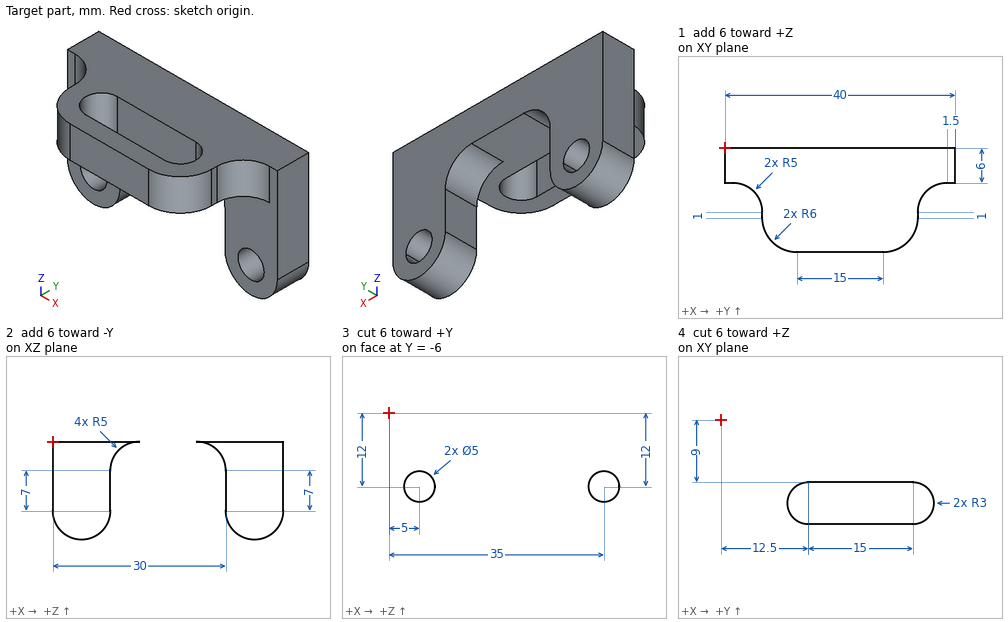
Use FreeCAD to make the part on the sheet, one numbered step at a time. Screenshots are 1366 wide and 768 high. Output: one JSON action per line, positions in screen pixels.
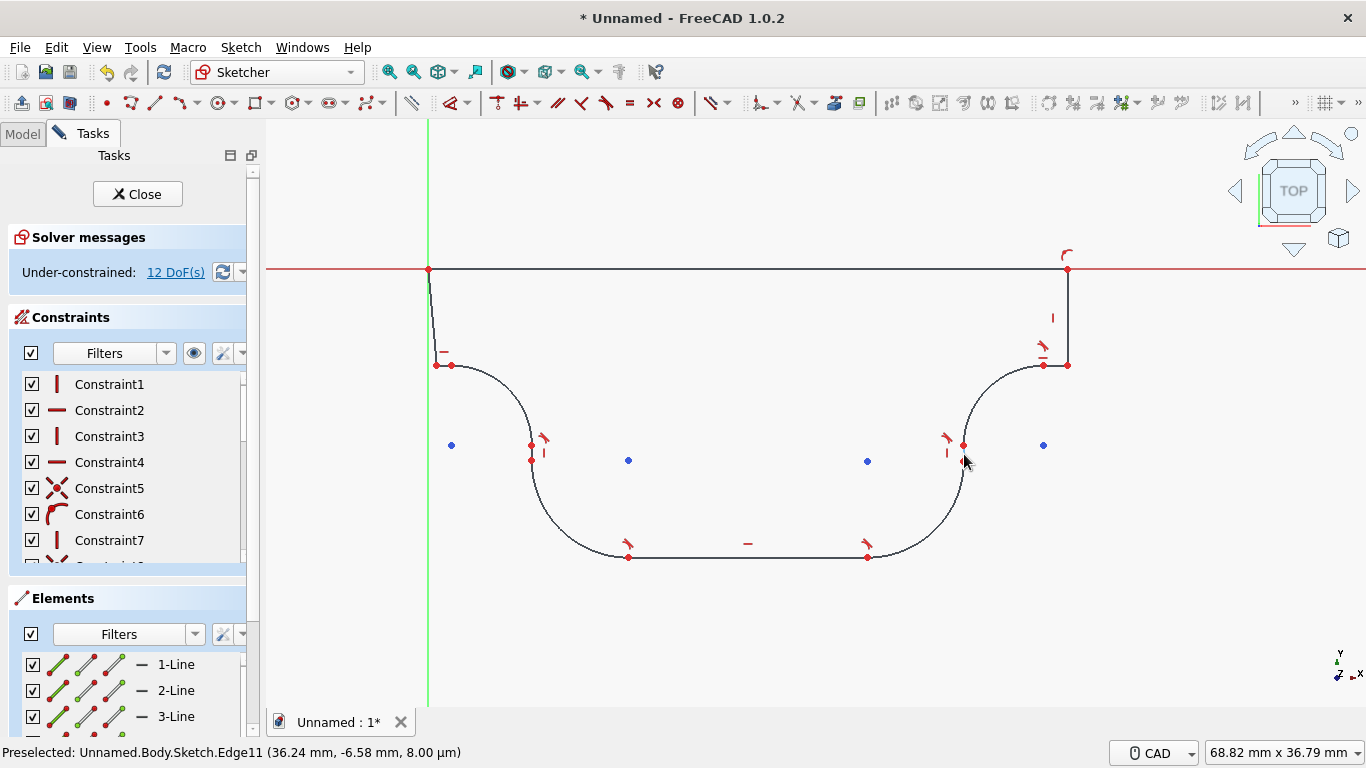
{"action": "scroll", "coordinate": [441, 366], "scroll_direction": "up", "scroll_amount": 6}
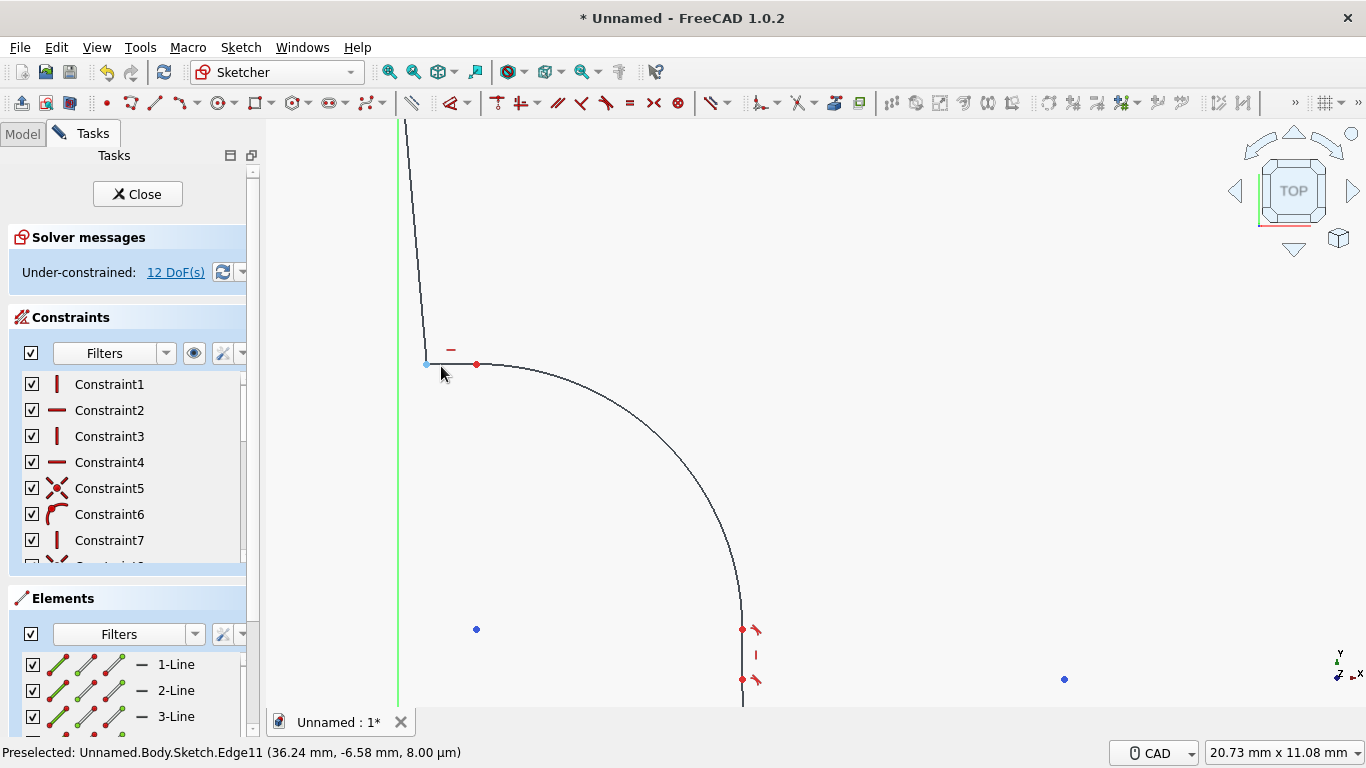
{"action": "left_click", "coordinate": [442, 364]}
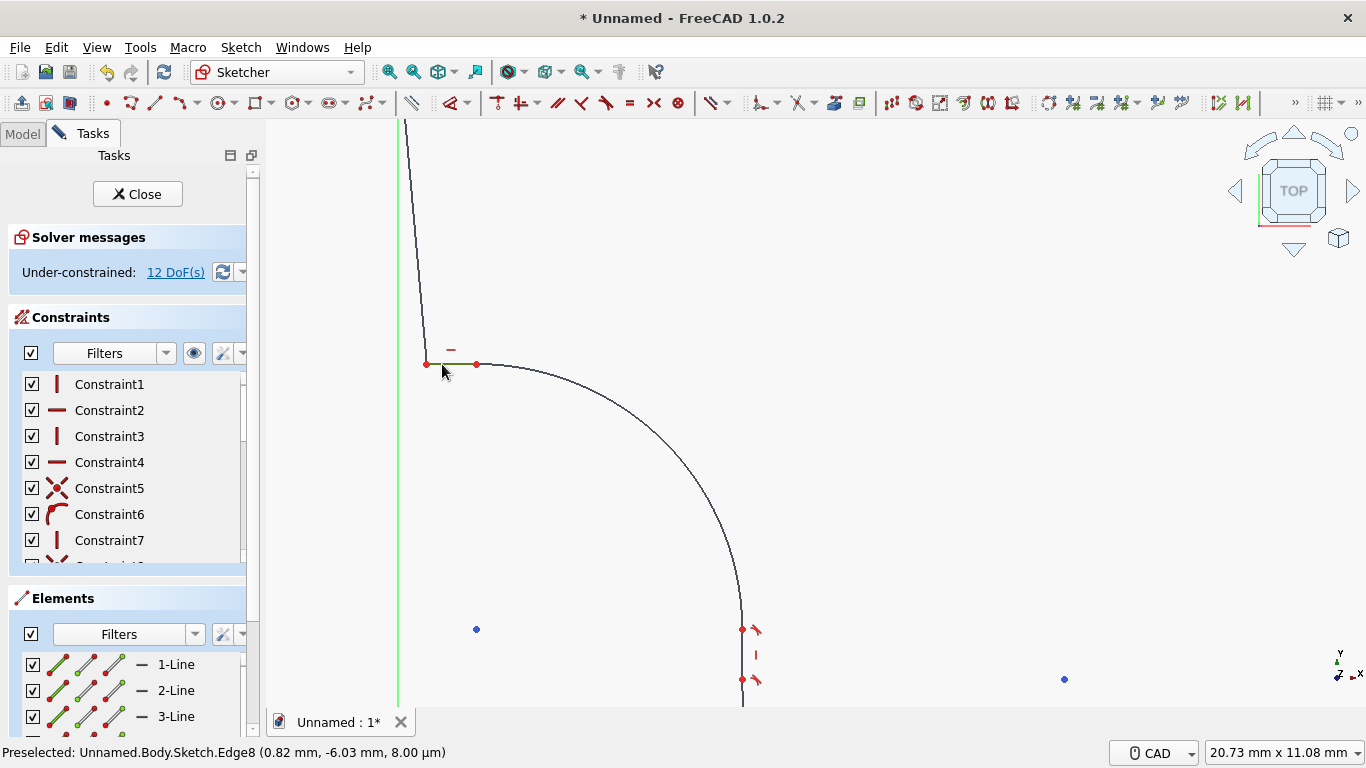
{"action": "left_click", "coordinate": [713, 509]}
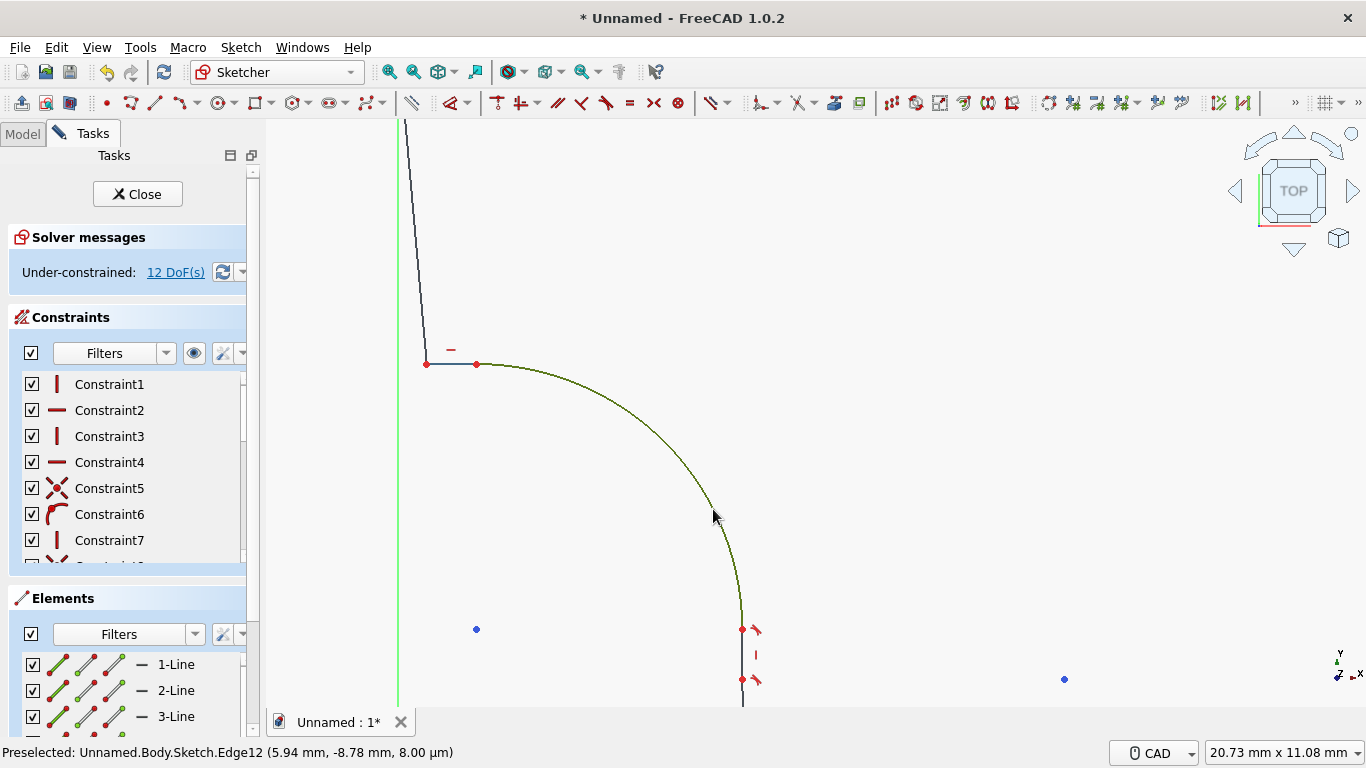
{"action": "left_click", "coordinate": [606, 104]}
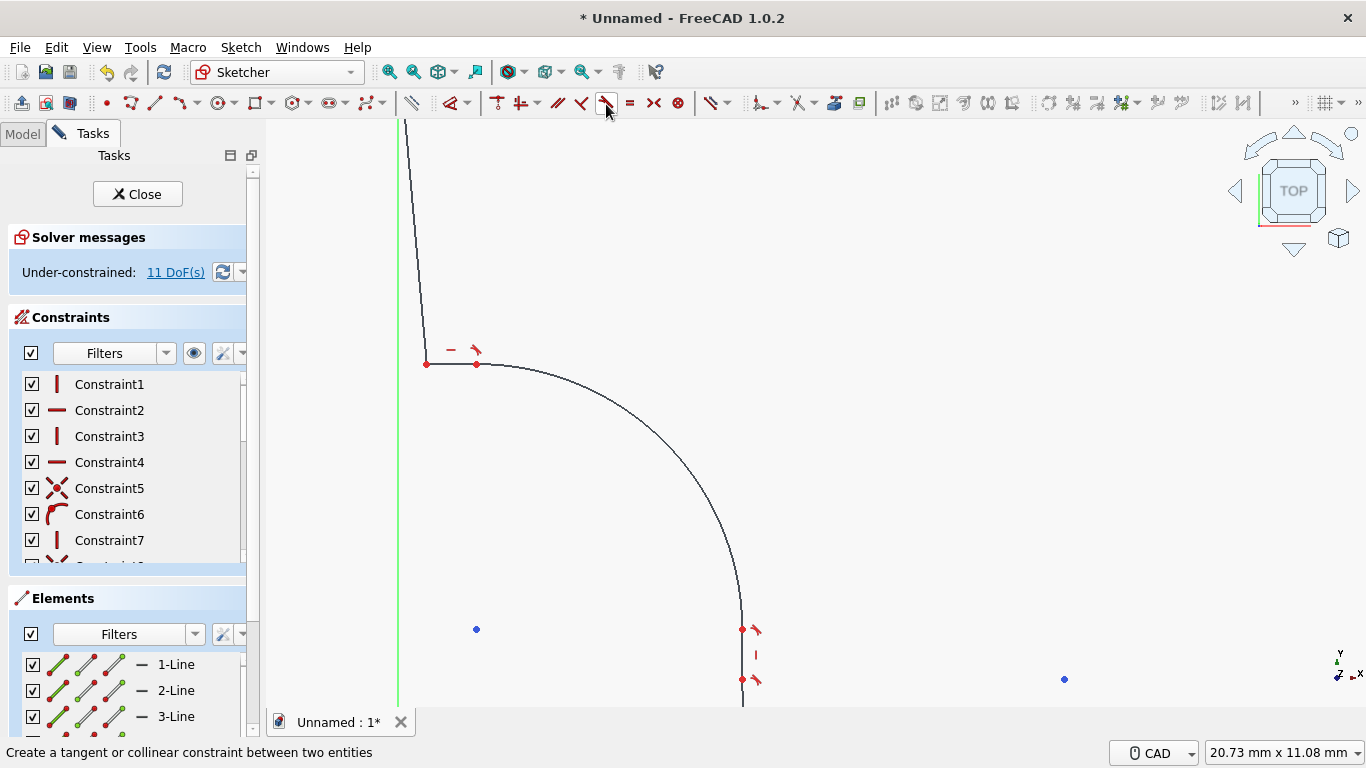
{"action": "left_click", "coordinate": [418, 268]}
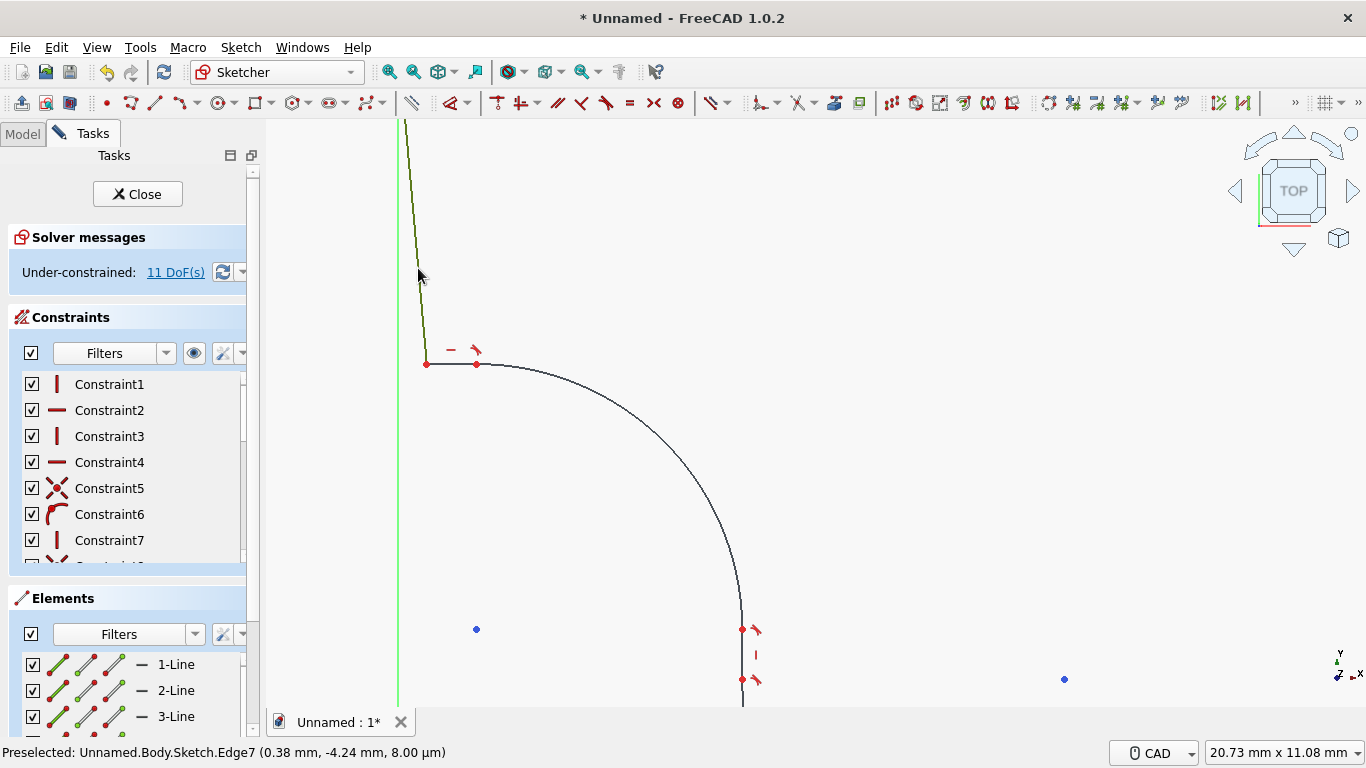
{"action": "key", "text": "v"}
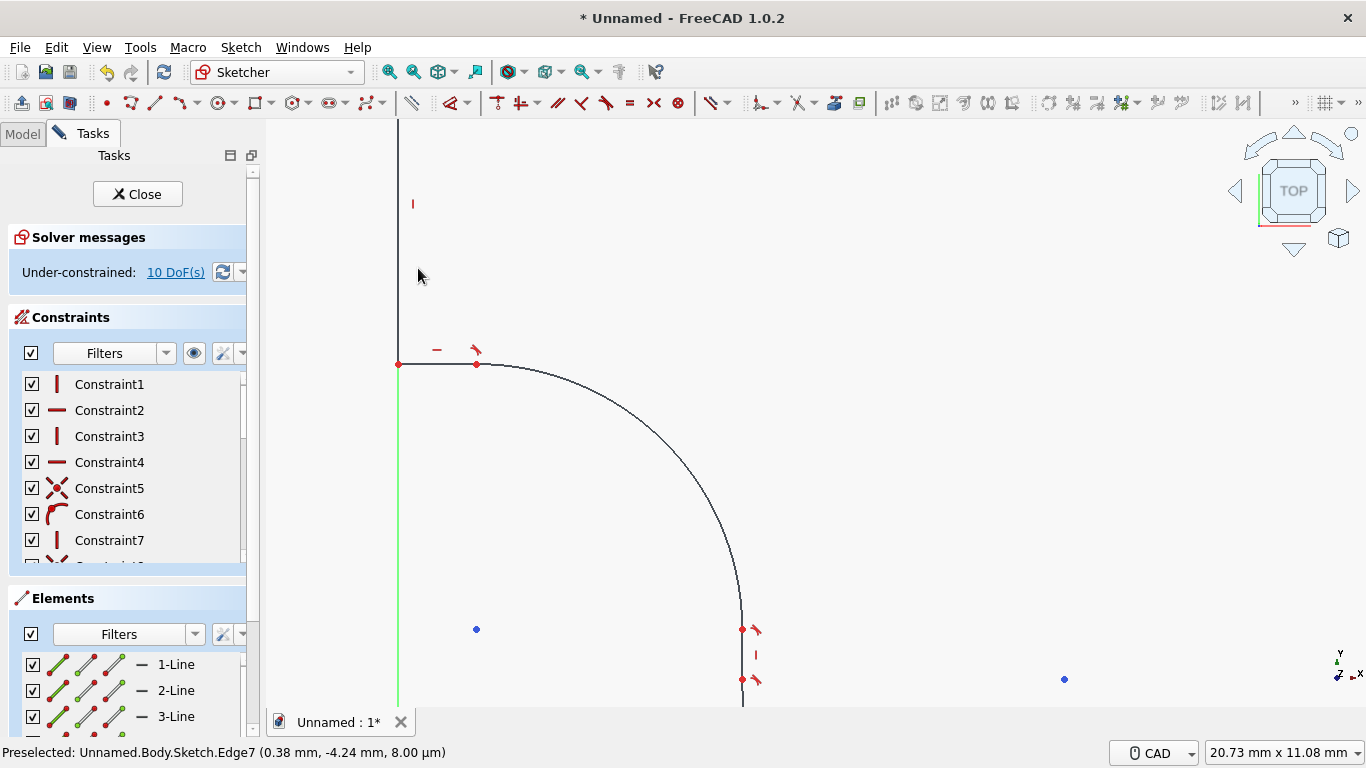
{"action": "scroll", "coordinate": [441, 366], "scroll_direction": "down", "scroll_amount": 6}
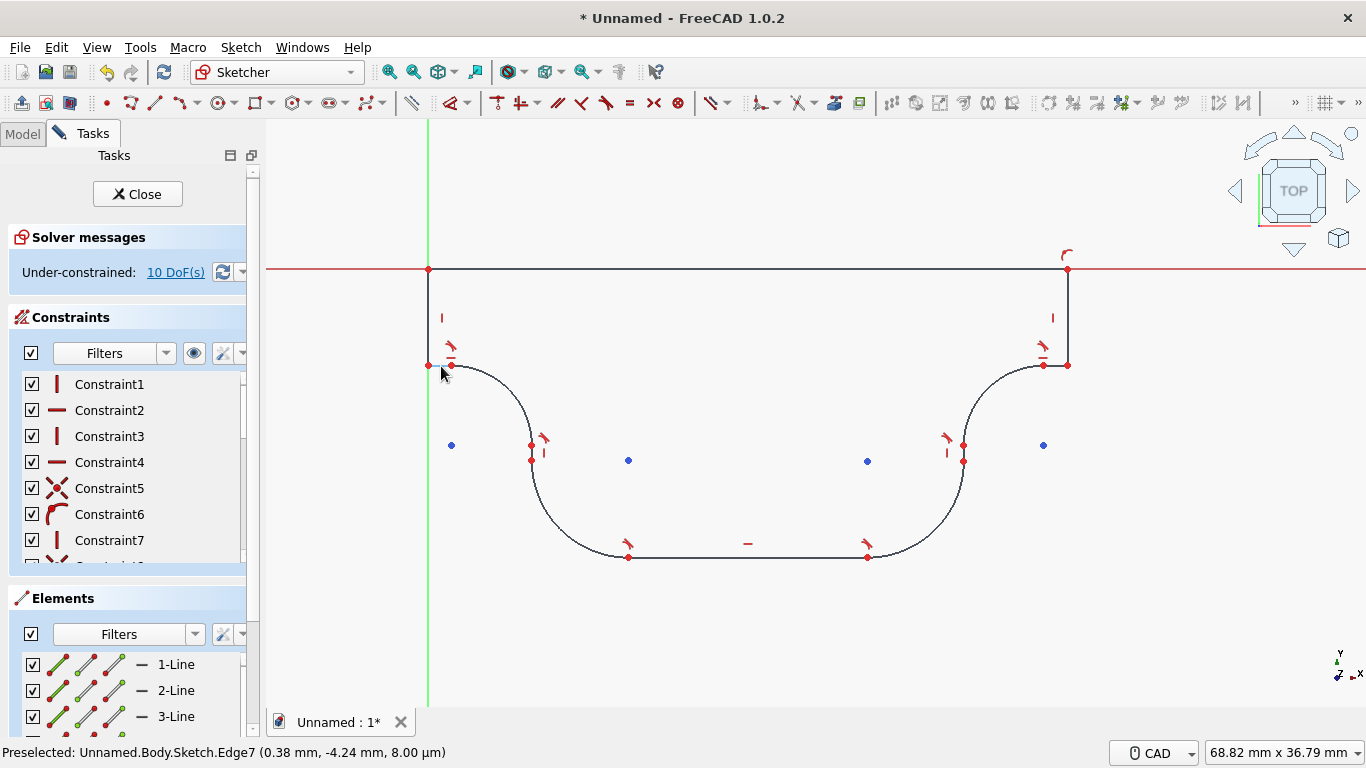
{"action": "left_click", "coordinate": [542, 505]}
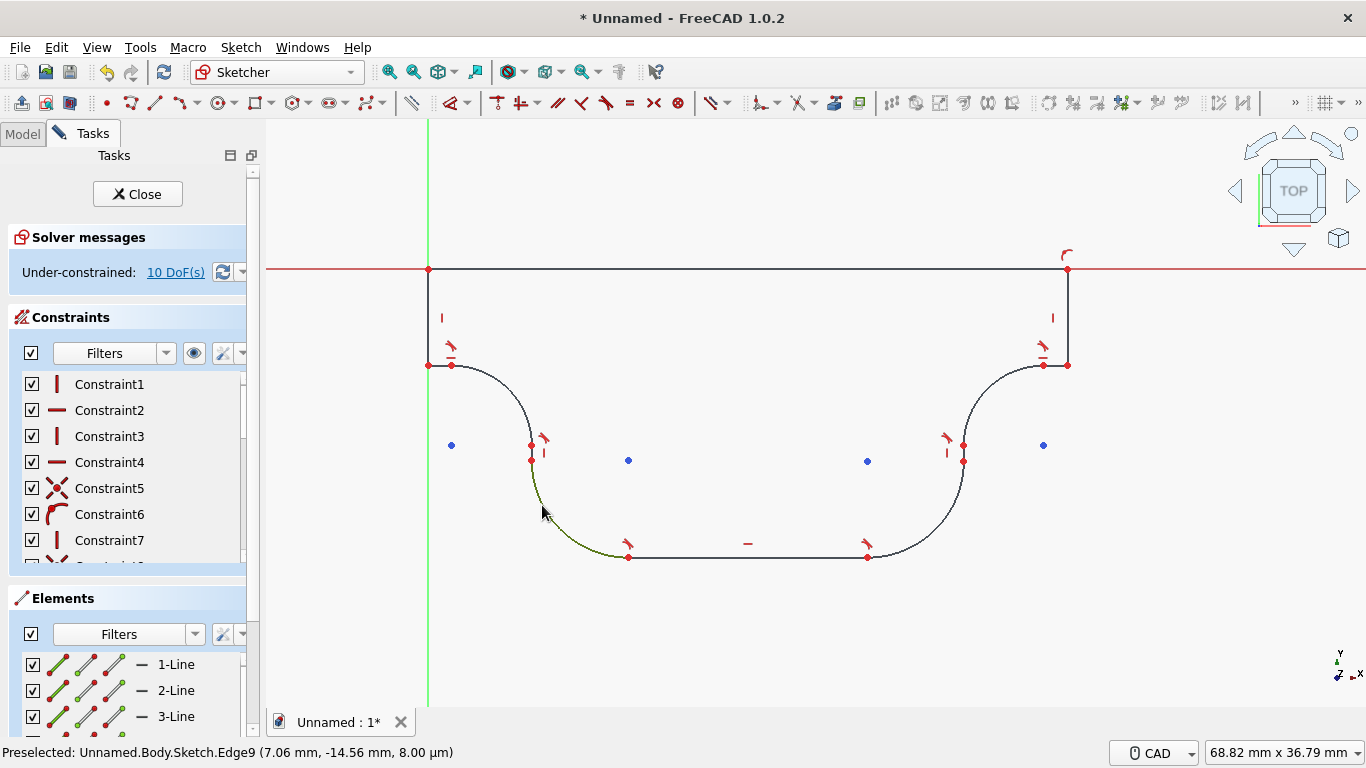
{"action": "left_click", "coordinate": [911, 547]}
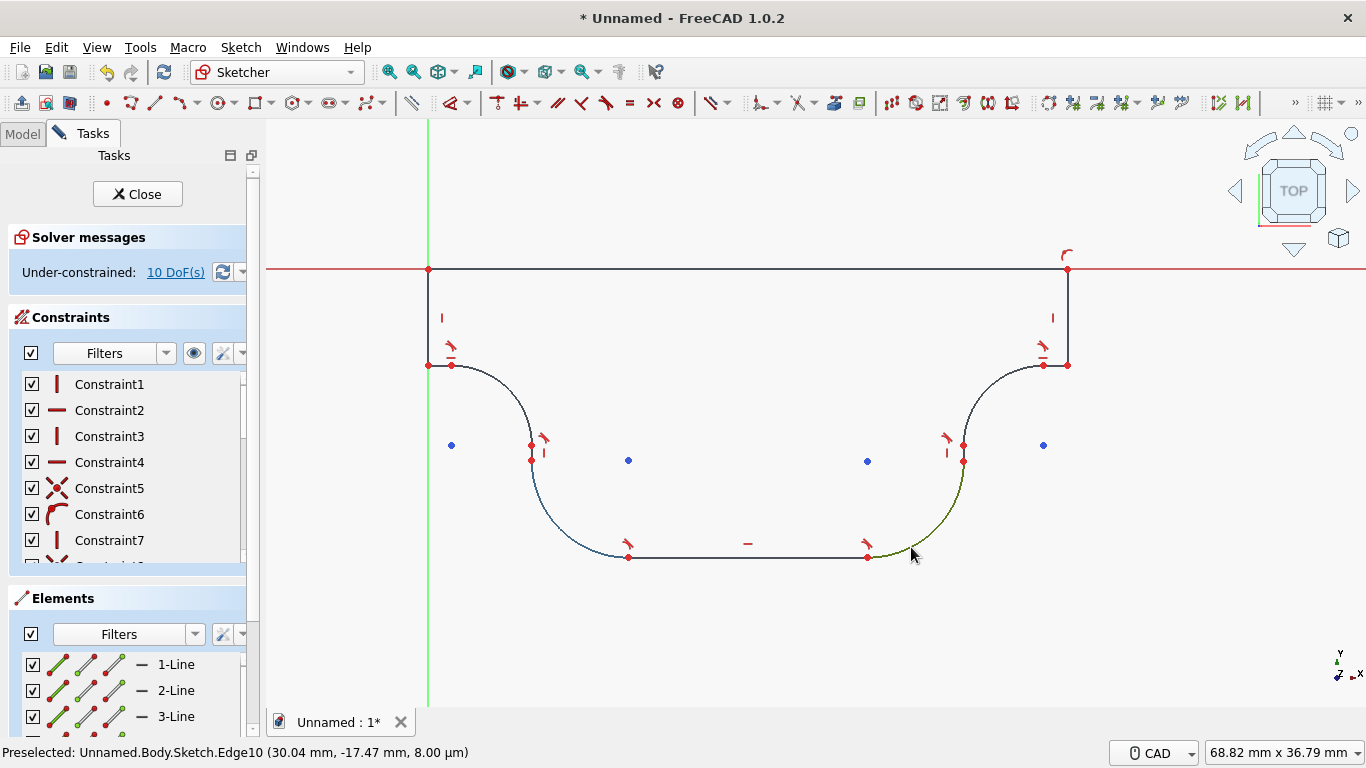
{"action": "left_click", "coordinate": [630, 104]}